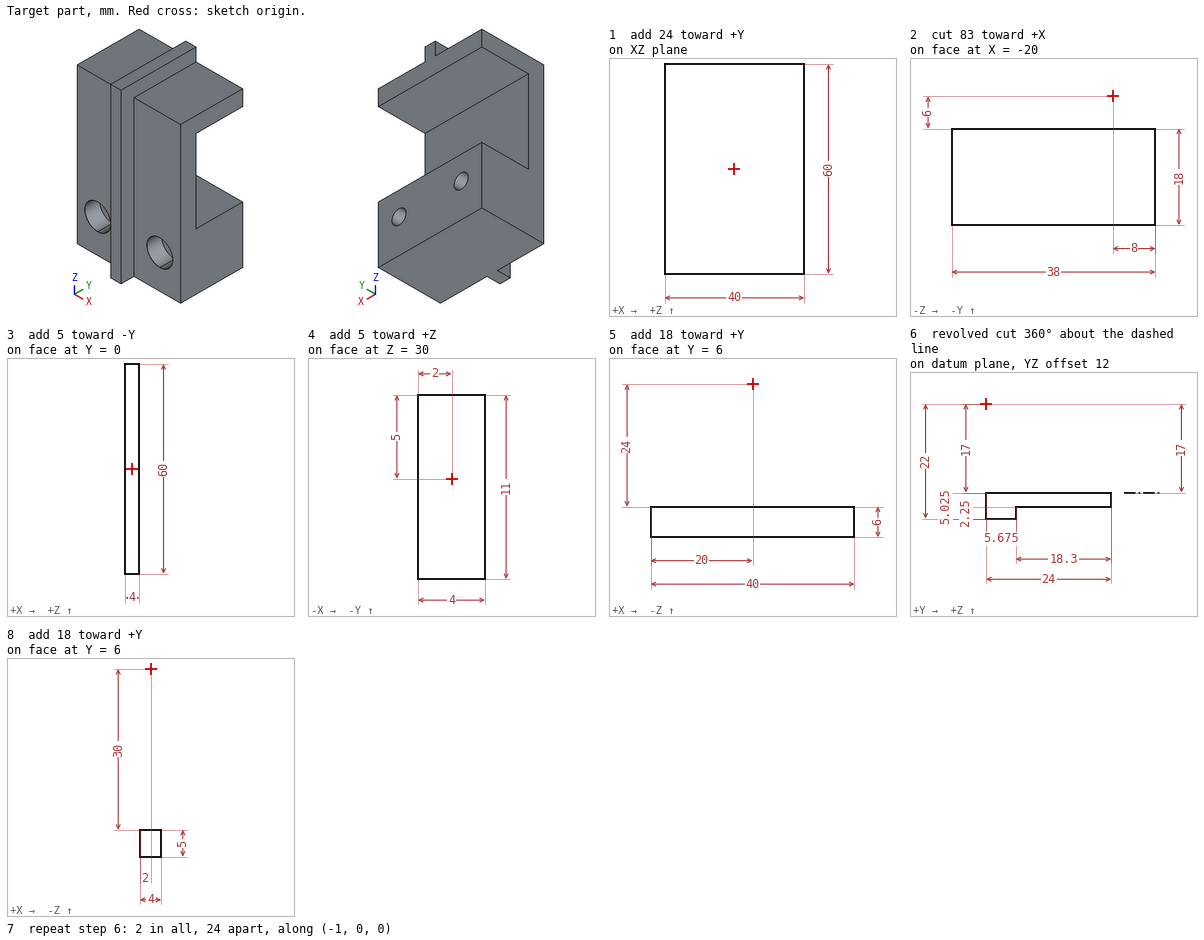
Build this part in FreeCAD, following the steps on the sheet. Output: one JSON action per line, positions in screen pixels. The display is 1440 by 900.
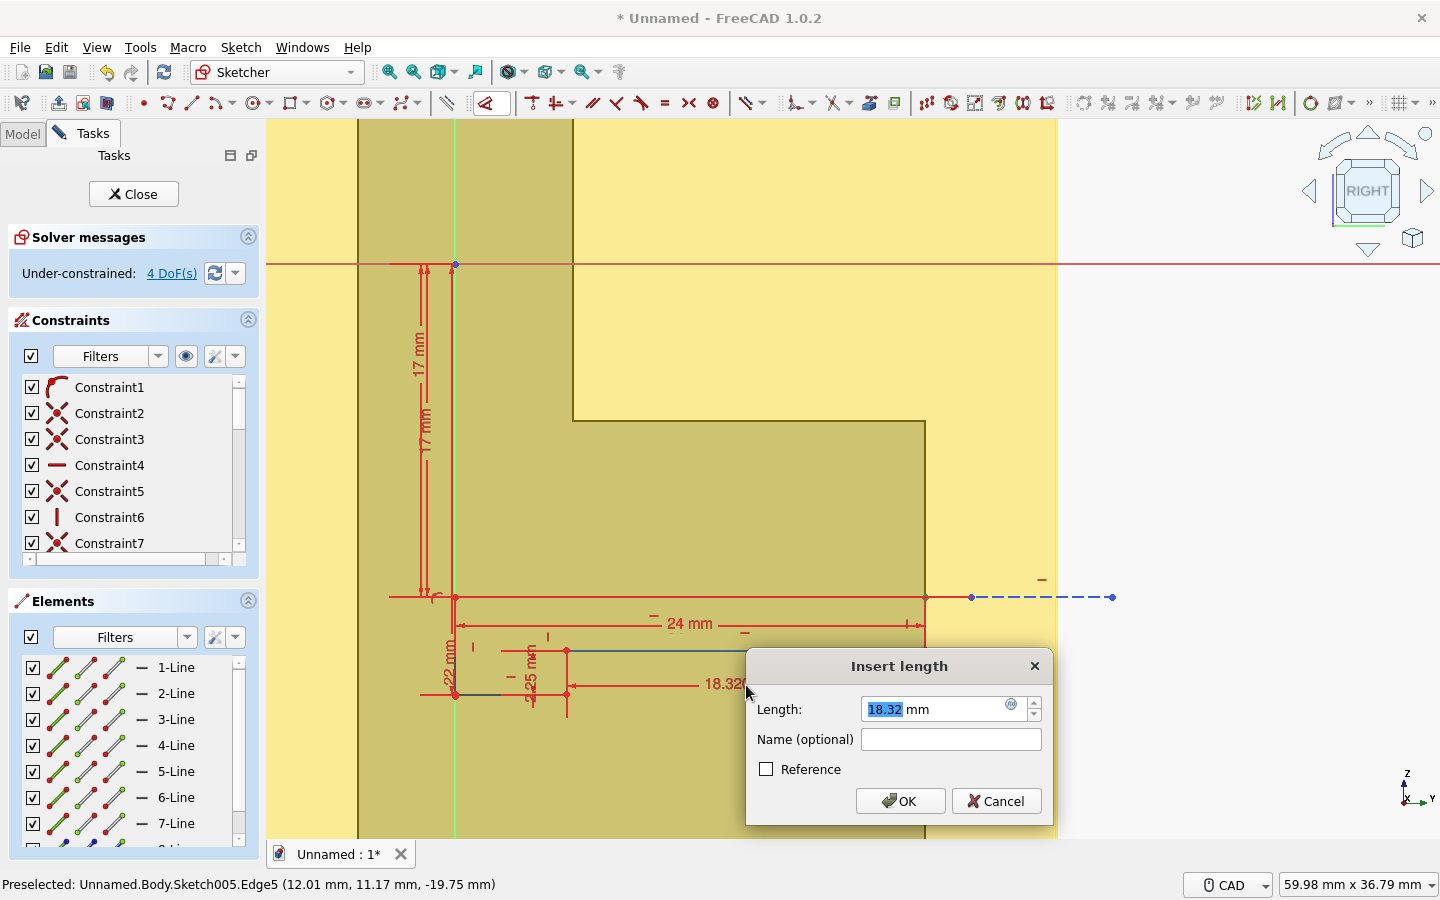
{"action": "type", "text": "18.3"}
{"action": "key", "text": "Return"}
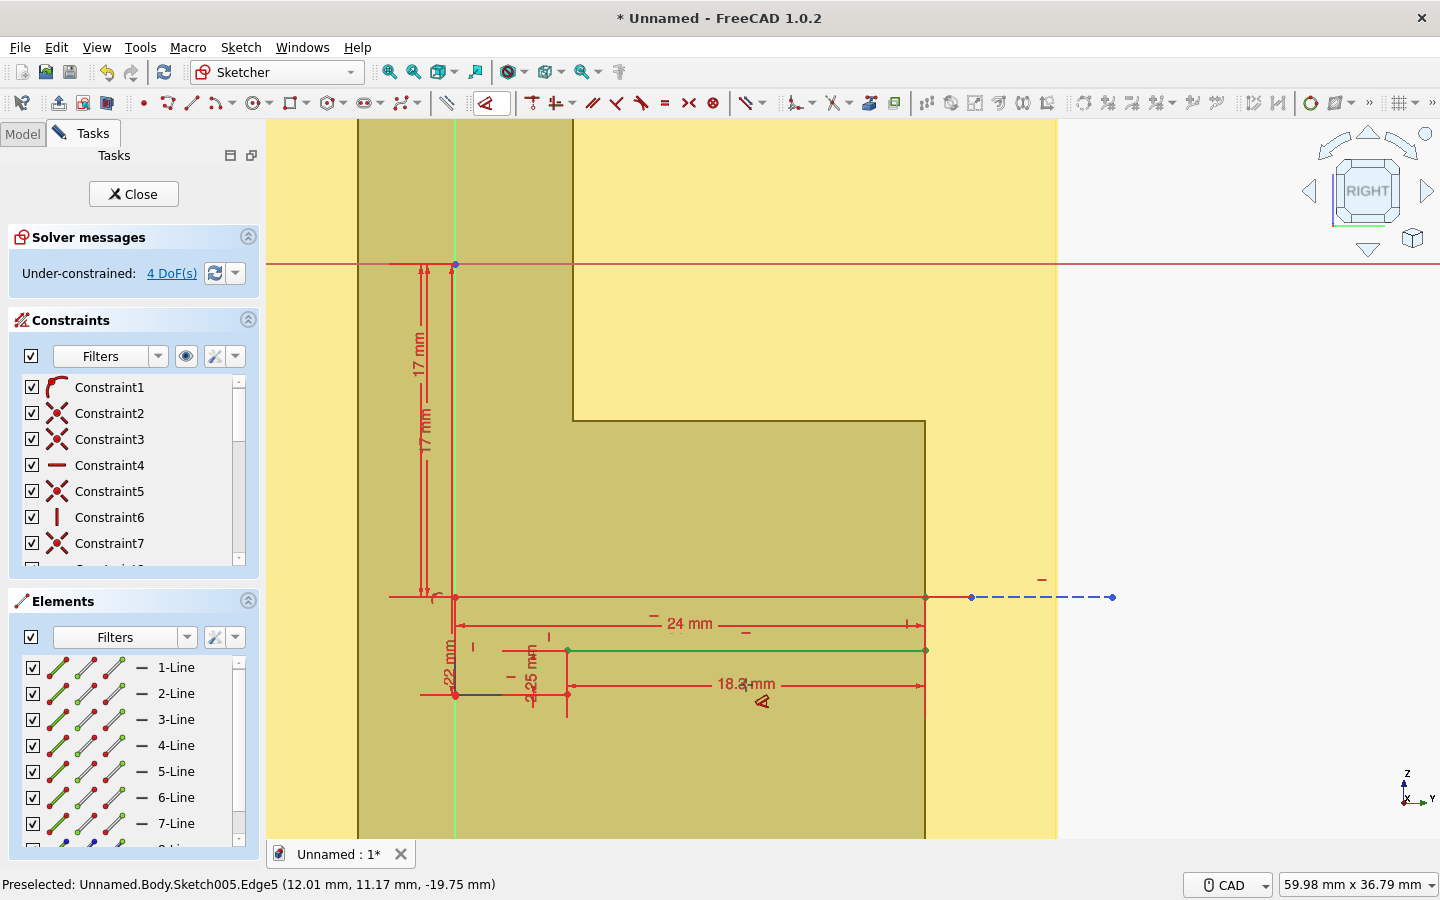
{"action": "left_click", "coordinate": [455, 627]}
{"action": "left_click", "coordinate": [421, 624]}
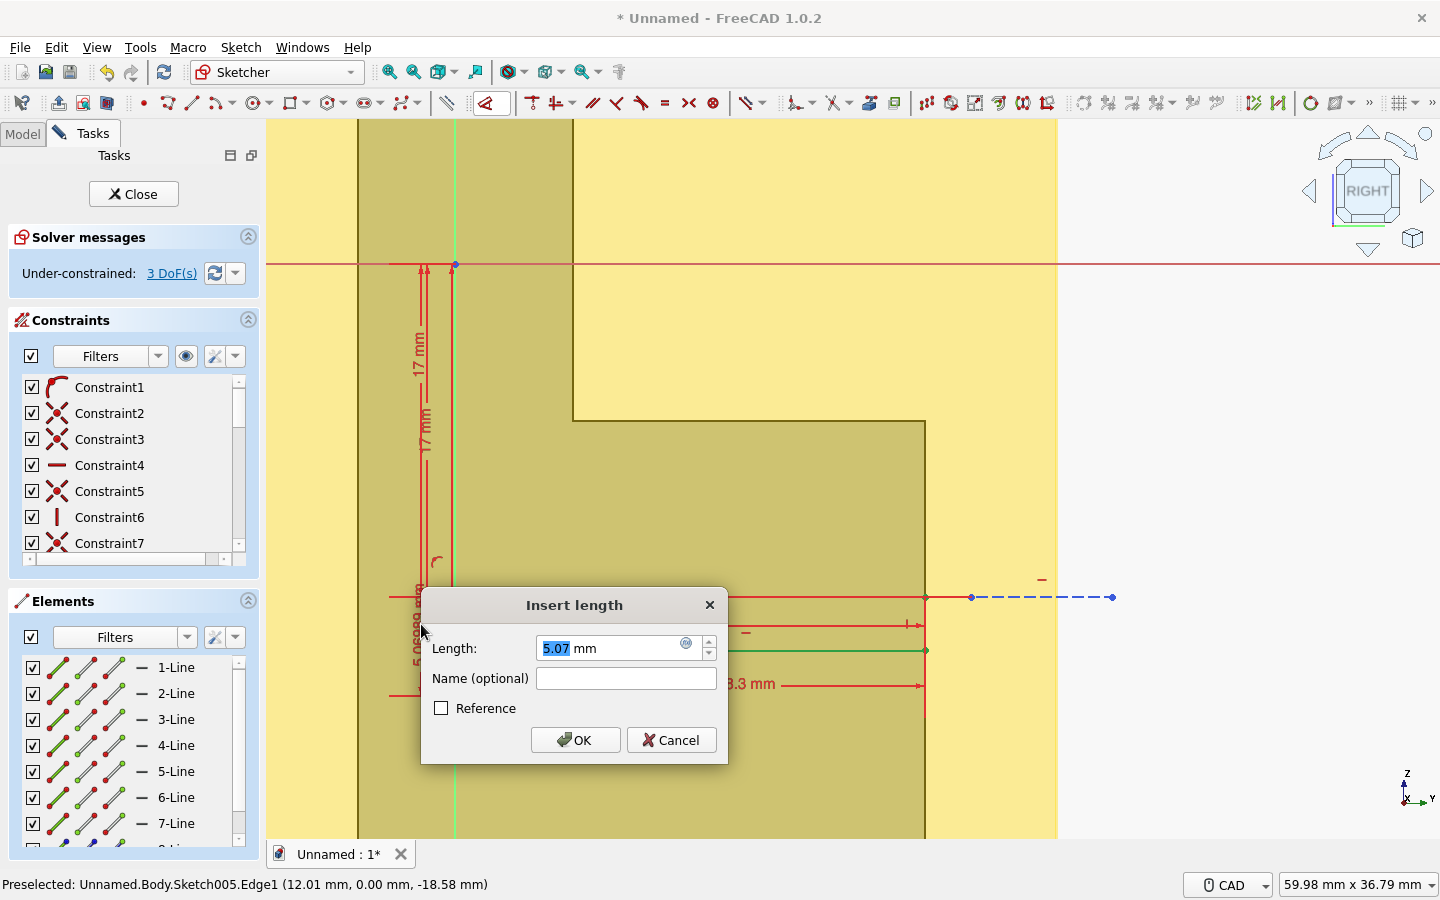
{"action": "type", "text": "5.025"}
{"action": "key", "text": "Return"}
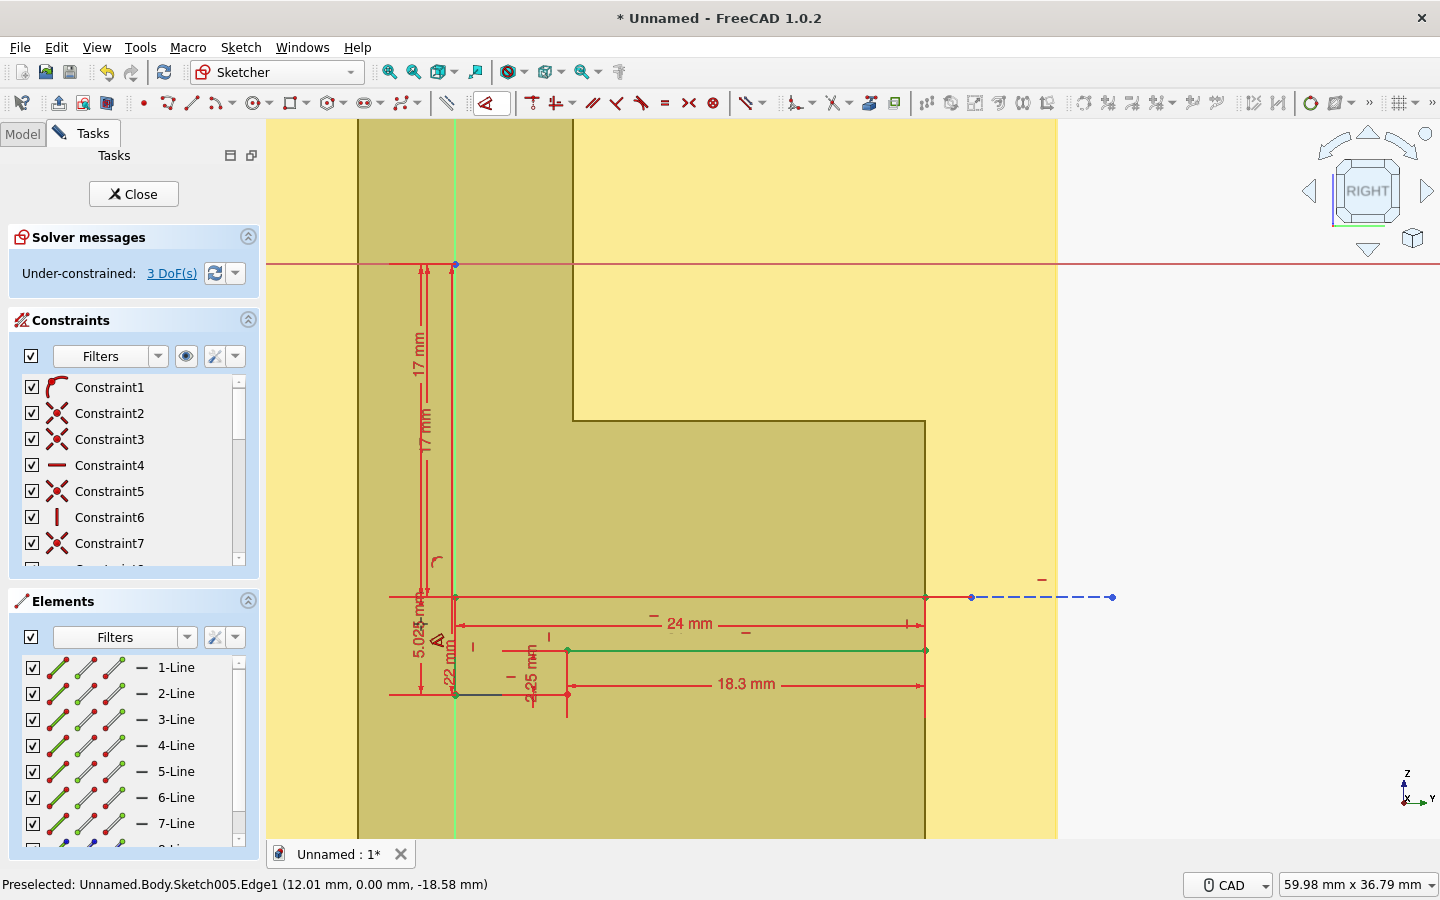
{"action": "left_click", "coordinate": [489, 695]}
{"action": "left_click", "coordinate": [511, 729]}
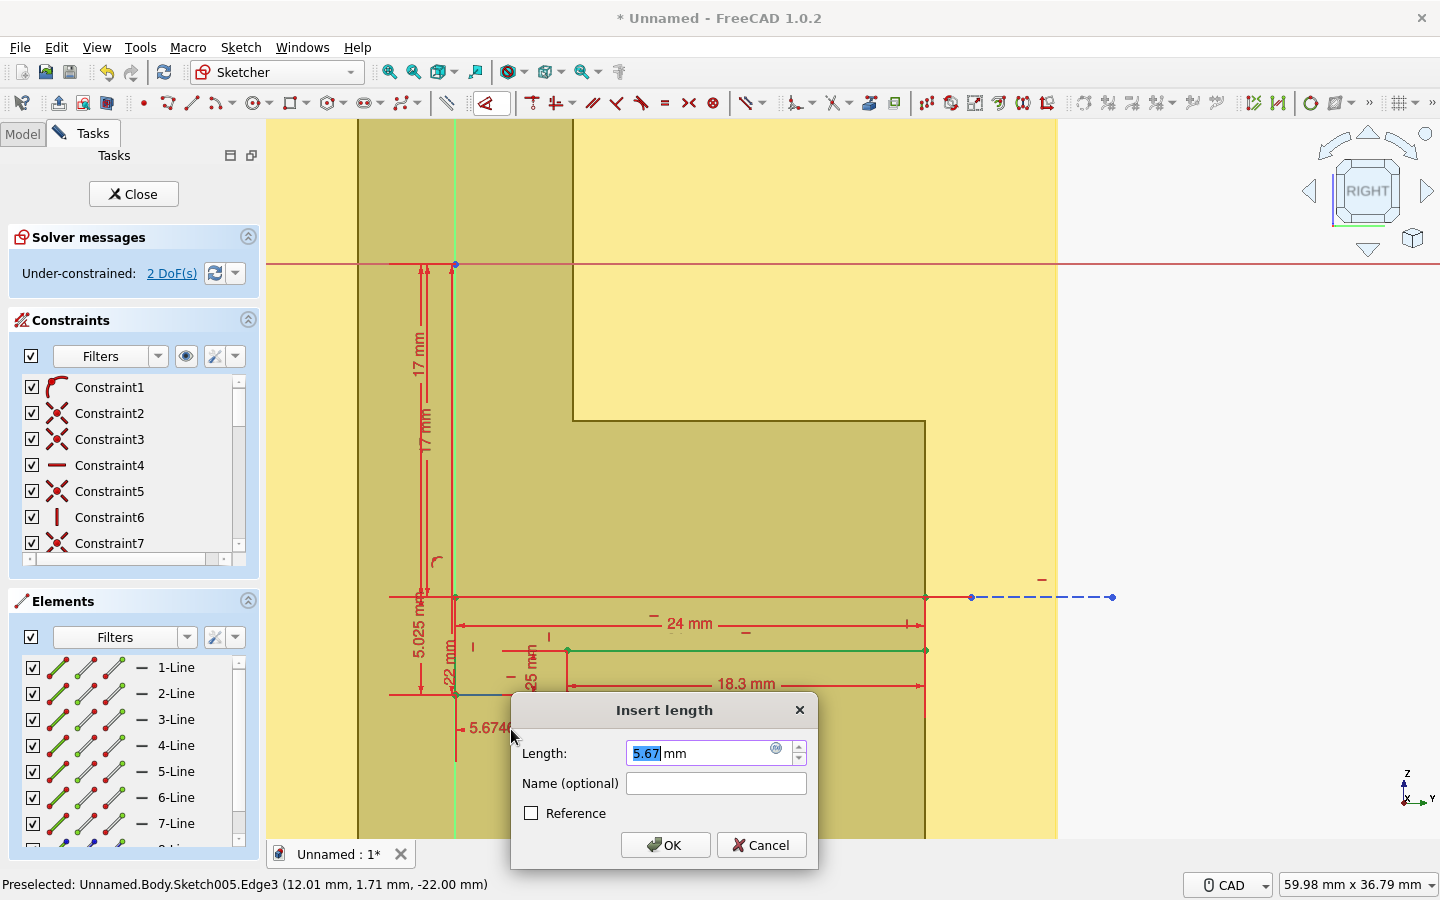
{"action": "type", "text": "5.675"}
{"action": "key", "text": "Return"}
{"action": "key", "text": "Escape"}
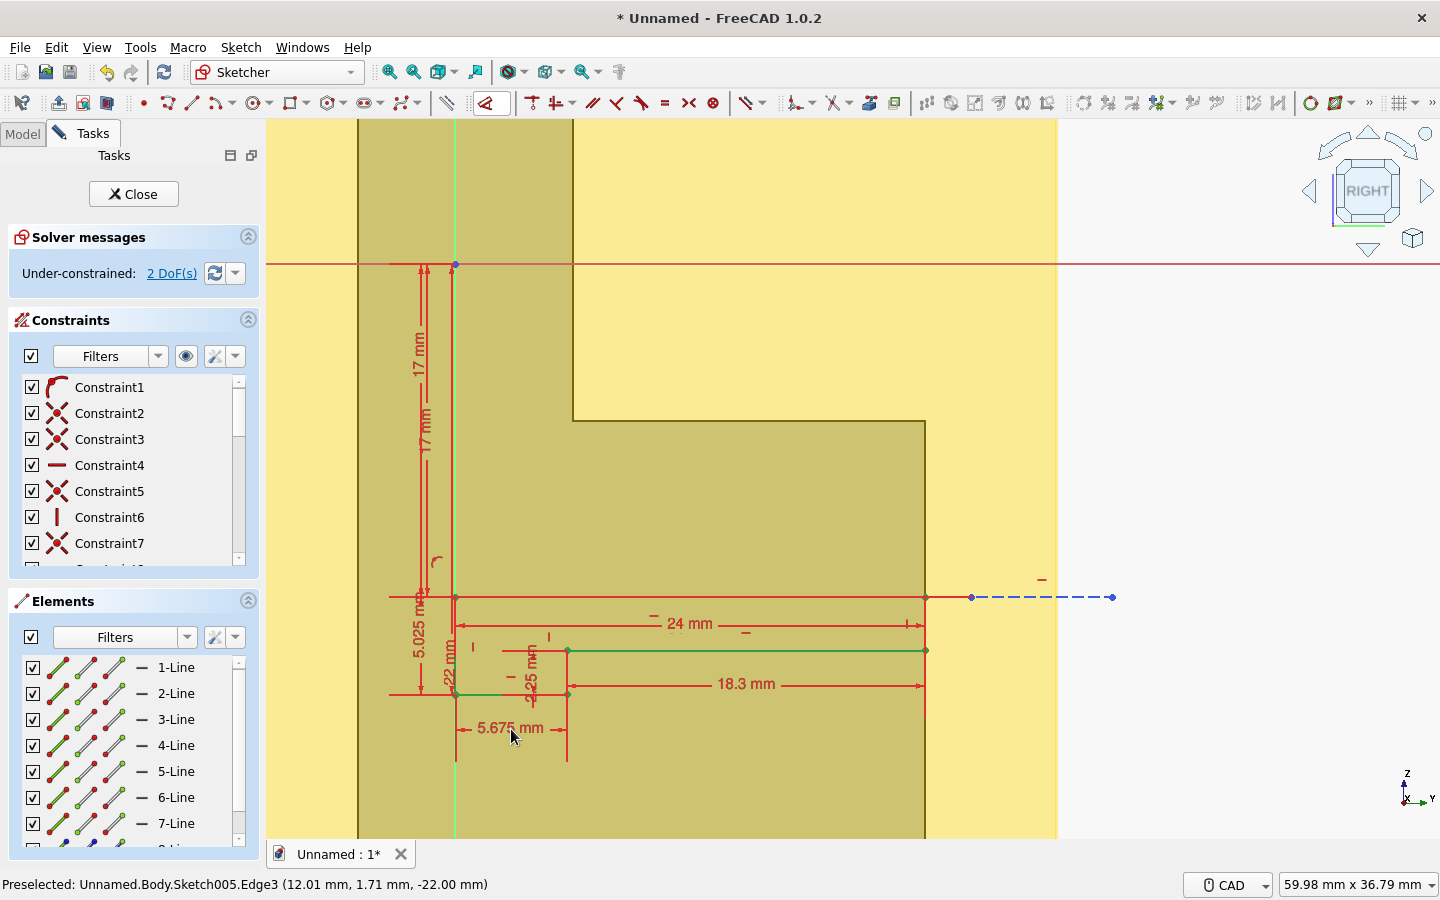
{"action": "left_click", "coordinate": [134, 194]}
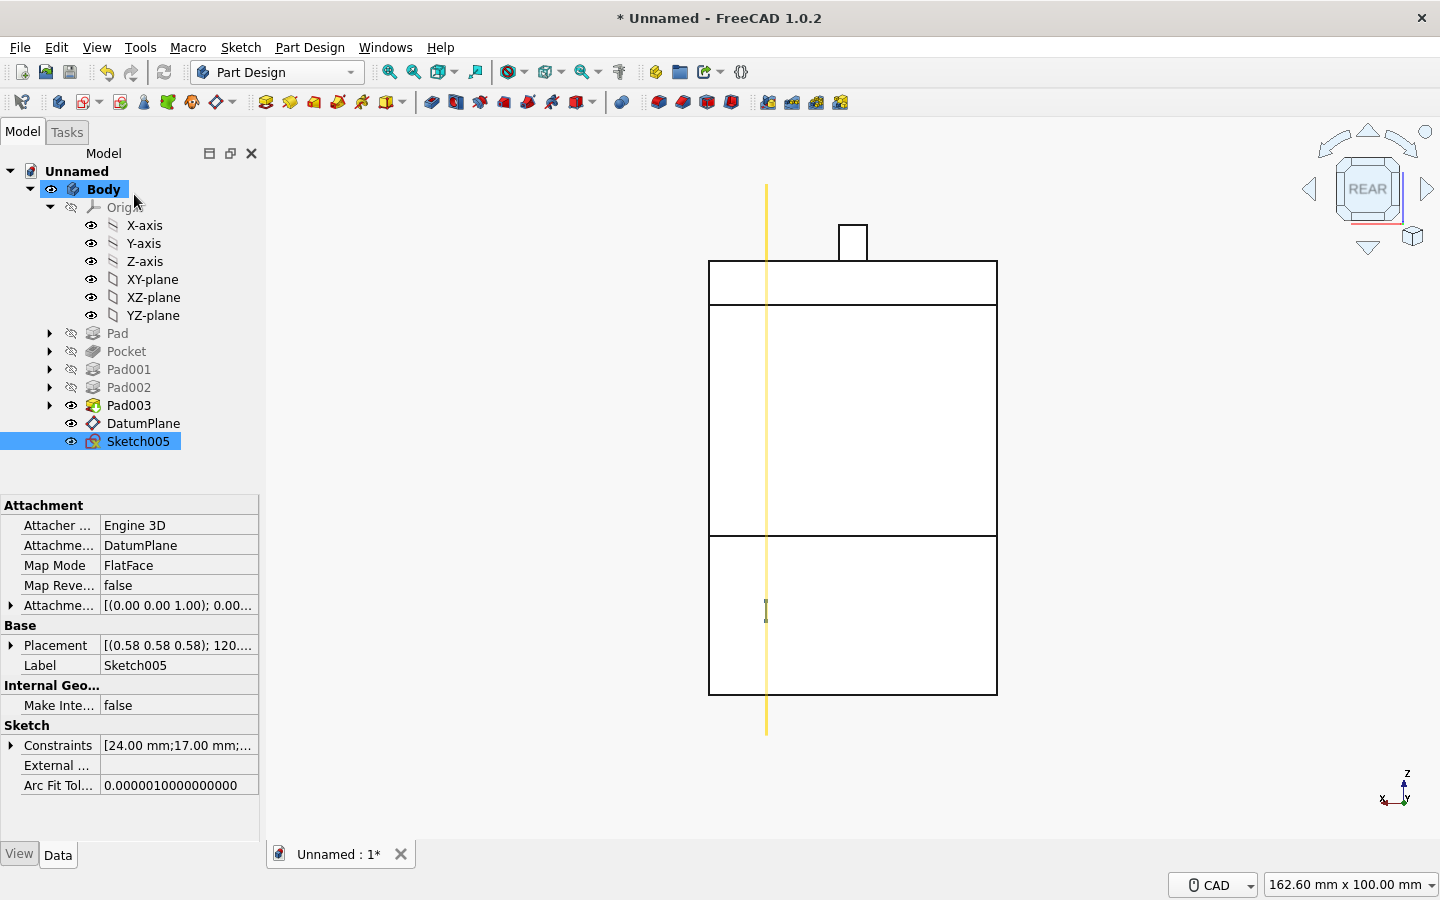
{"action": "left_click", "coordinate": [480, 102]}